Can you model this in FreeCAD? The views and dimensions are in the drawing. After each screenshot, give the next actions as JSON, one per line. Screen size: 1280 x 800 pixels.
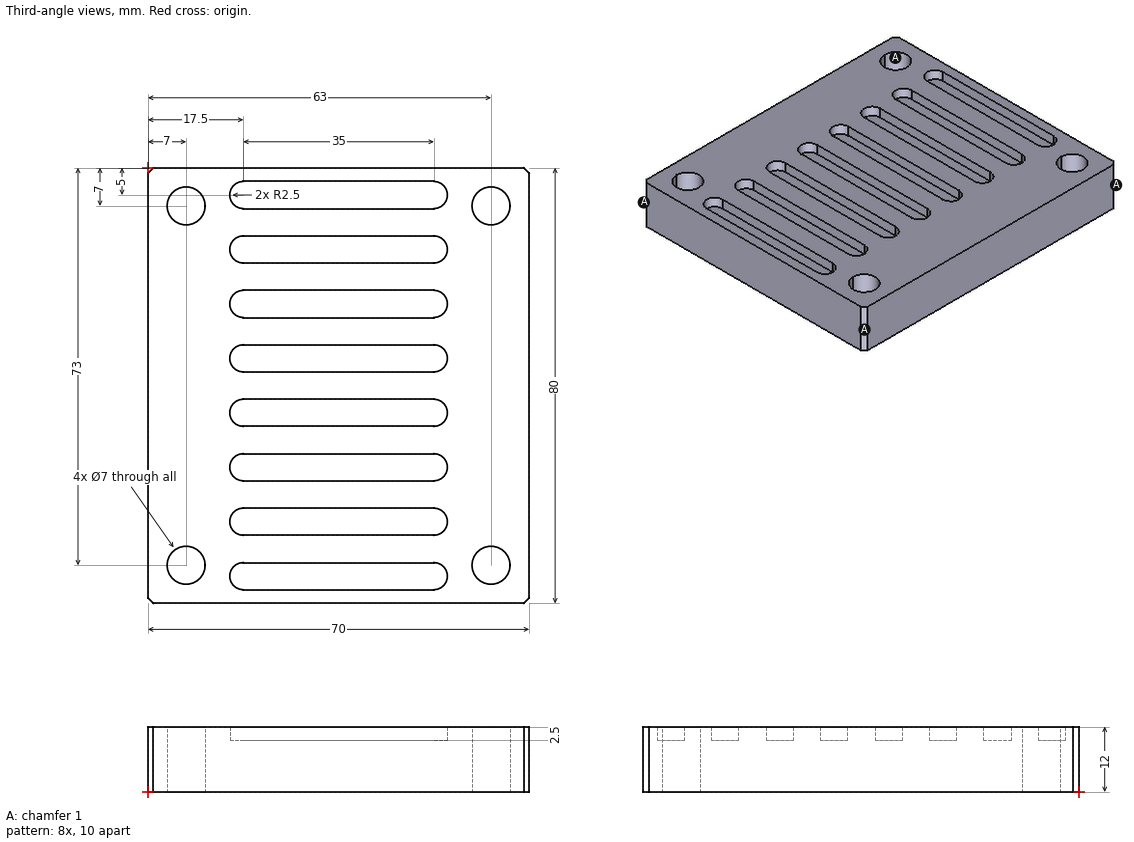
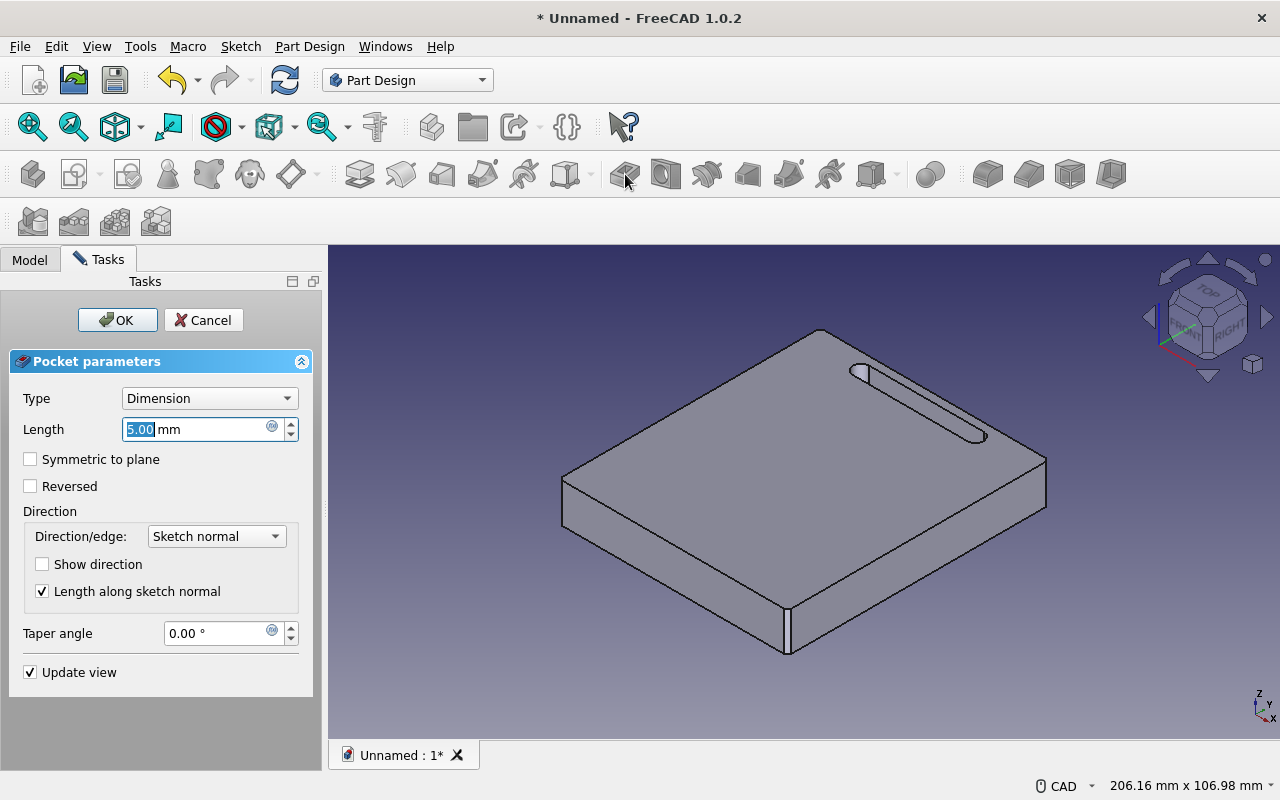
{"action": "type", "text": "2.5"}
{"action": "key", "text": "Tab"}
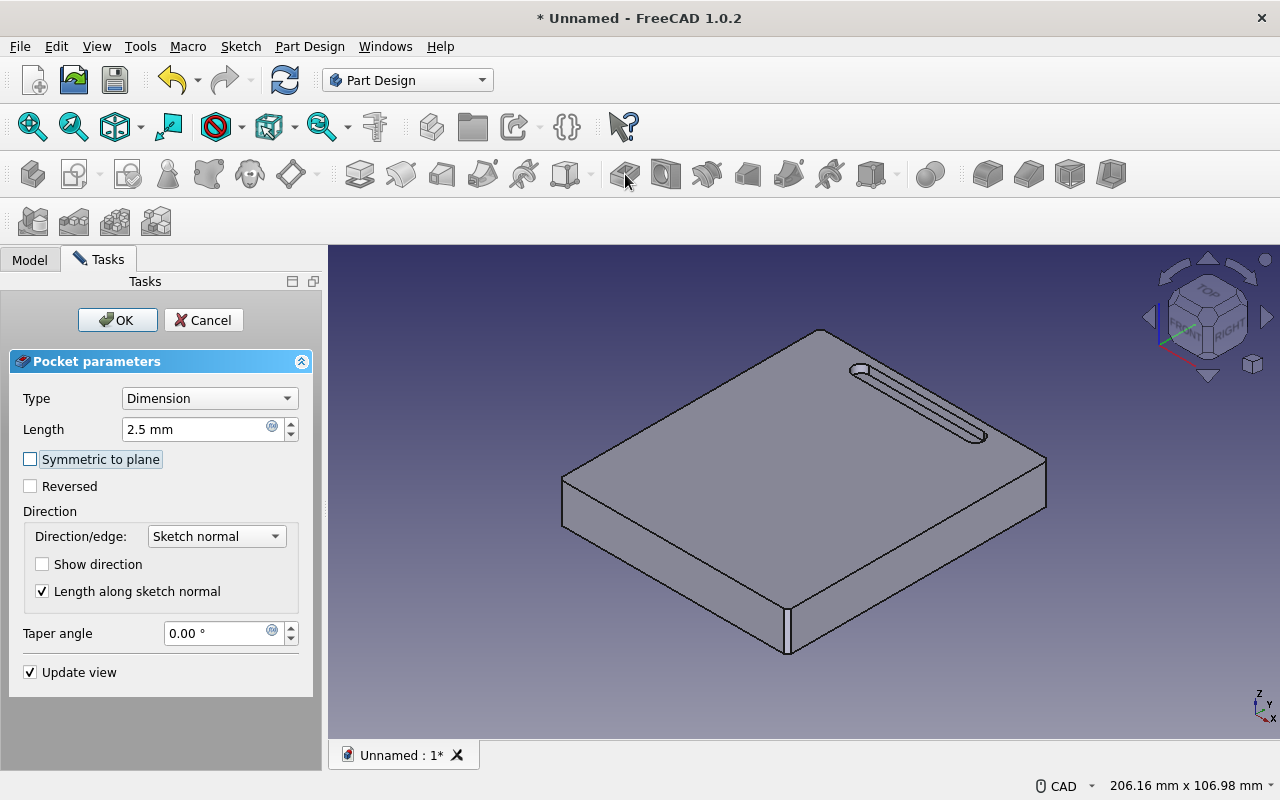
{"action": "left_click", "coordinate": [118, 320]}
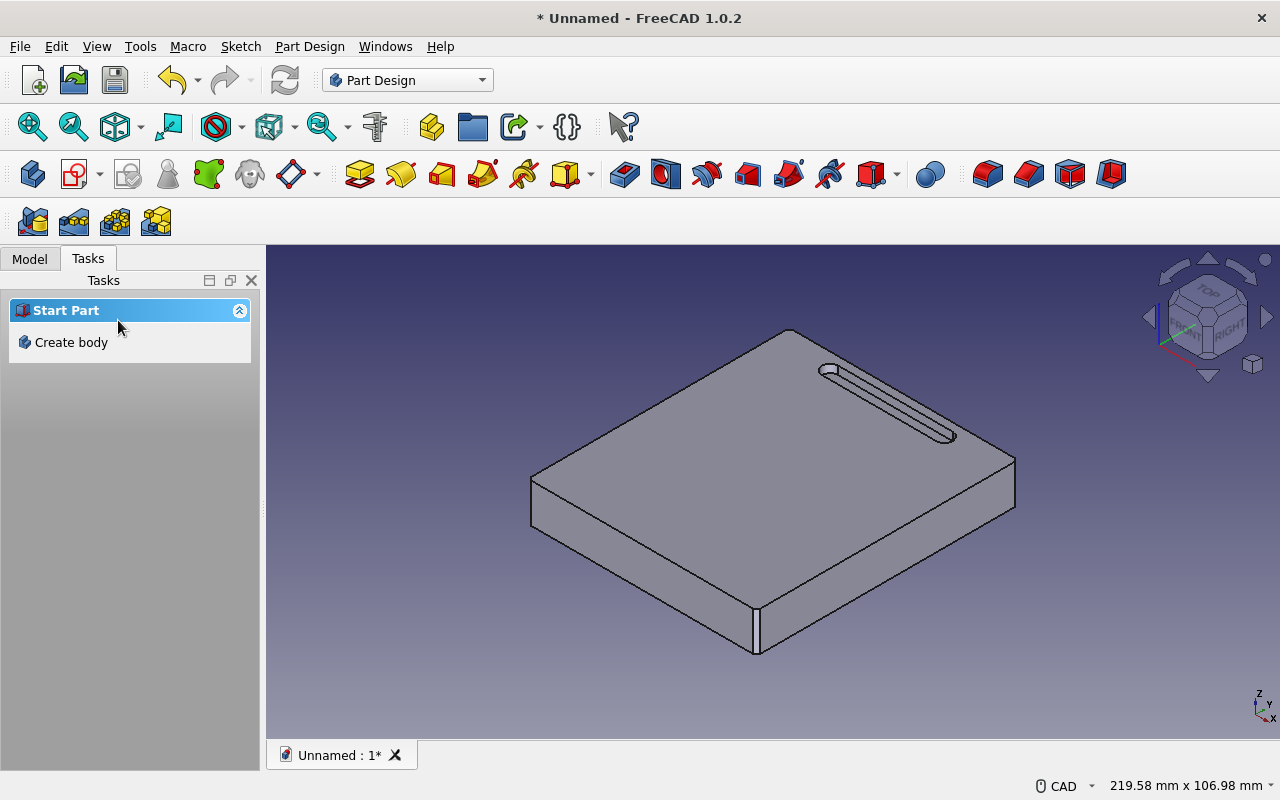
{"action": "left_click", "coordinate": [30, 258]}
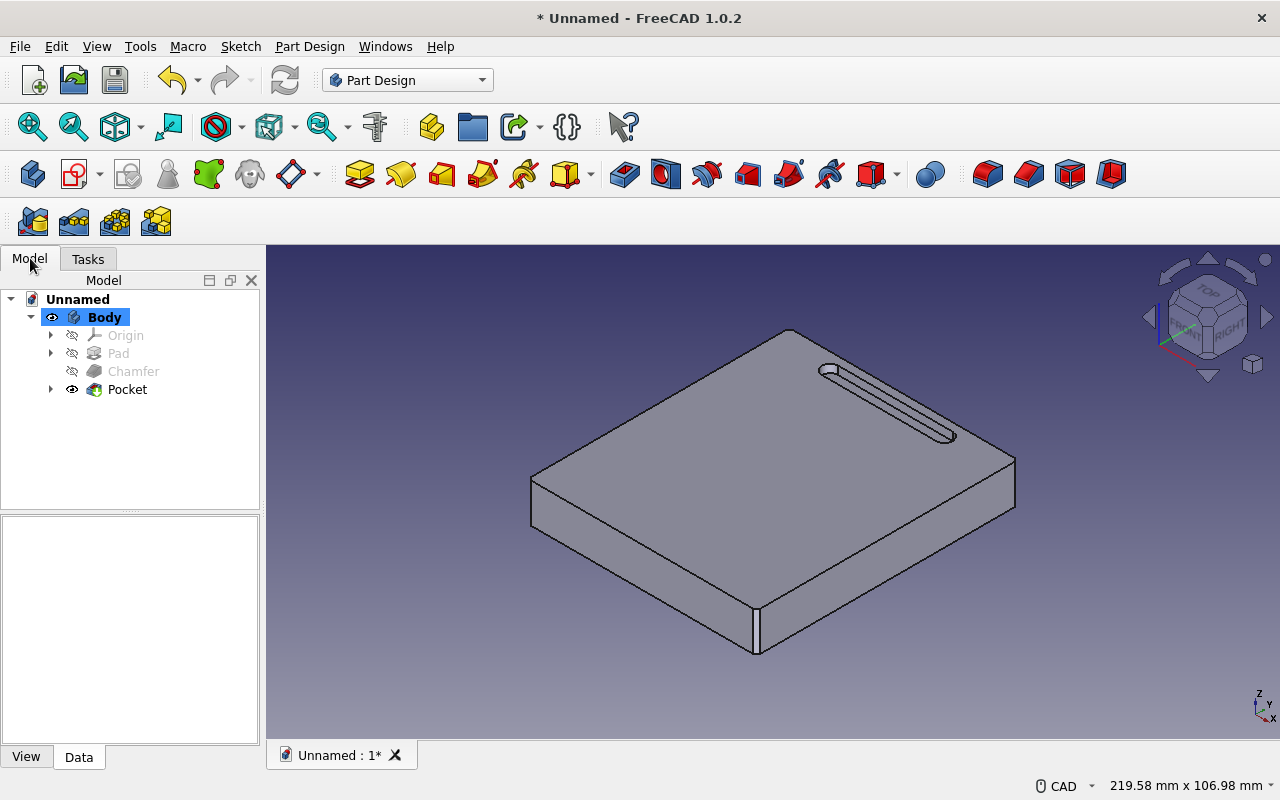
{"action": "left_click", "coordinate": [117, 389]}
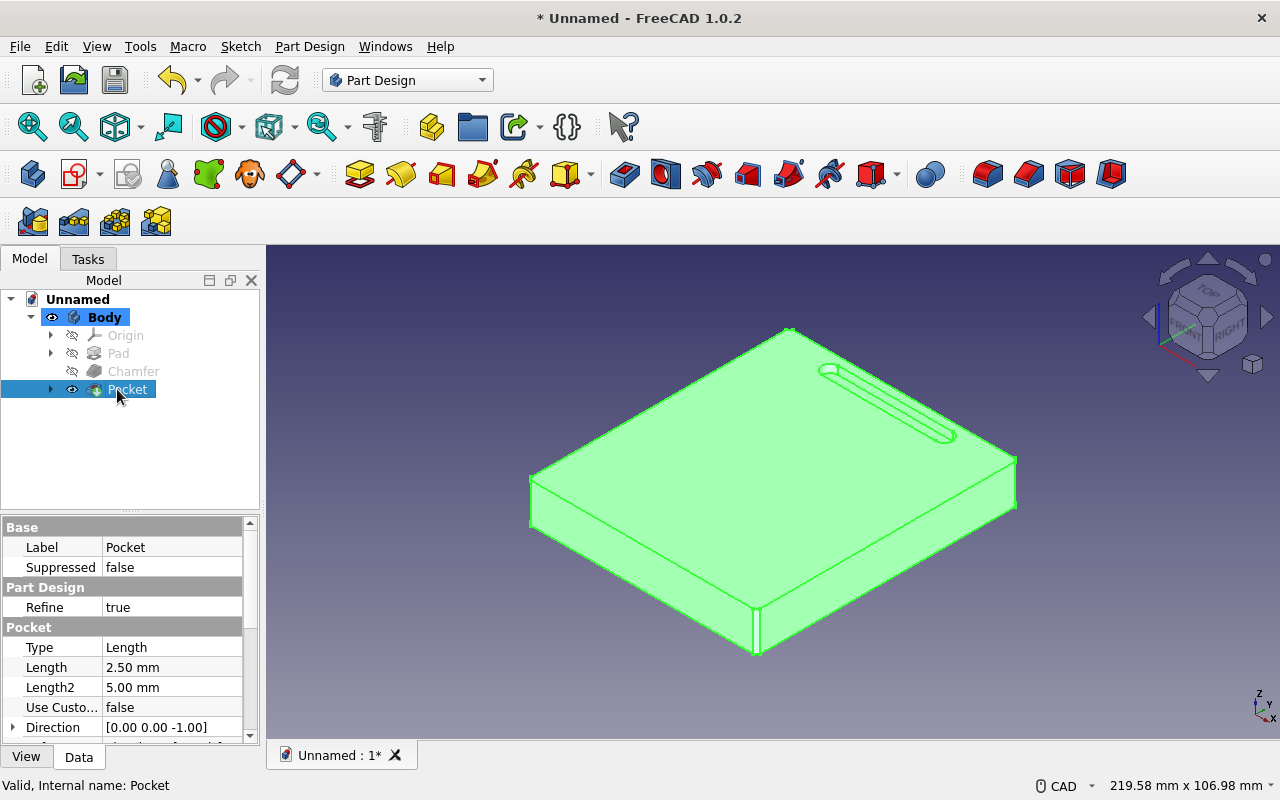
{"action": "left_click", "coordinate": [74, 222]}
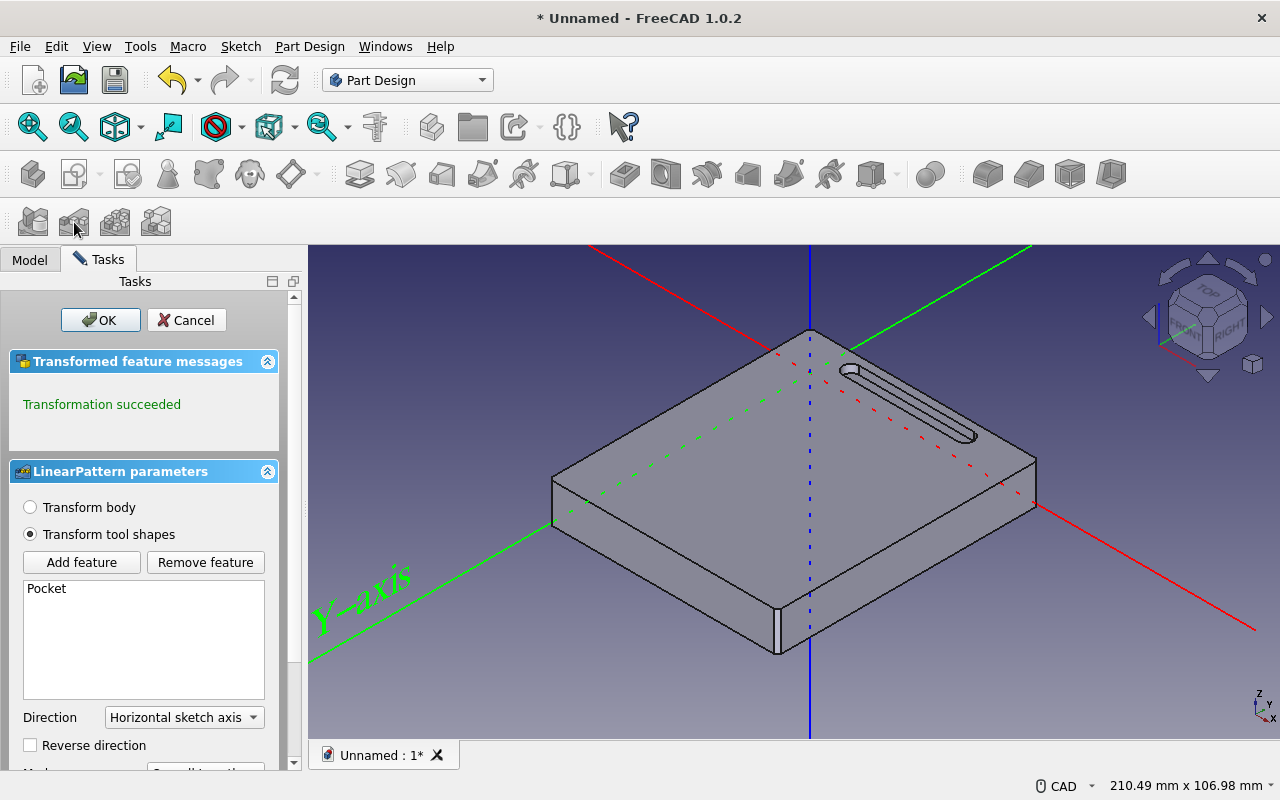
{"action": "left_click", "coordinate": [185, 718]}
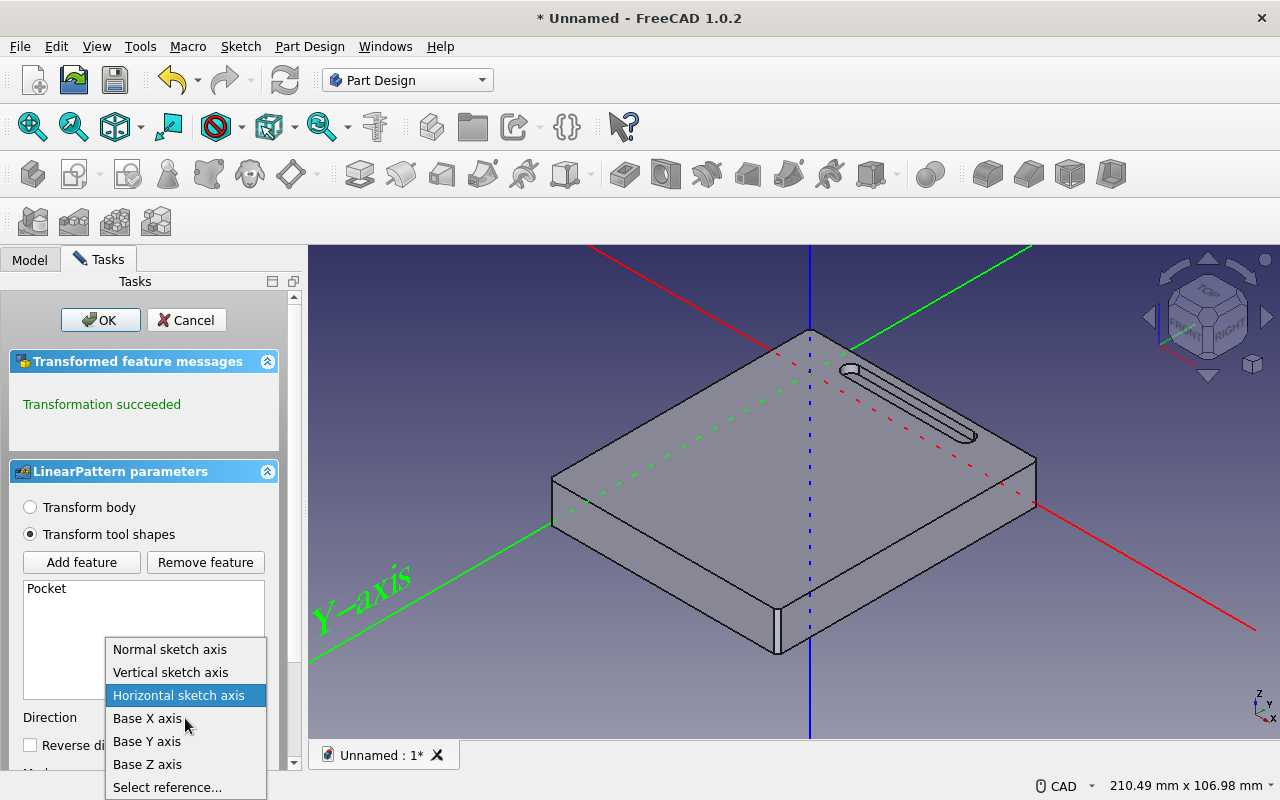
{"action": "left_click", "coordinate": [184, 742]}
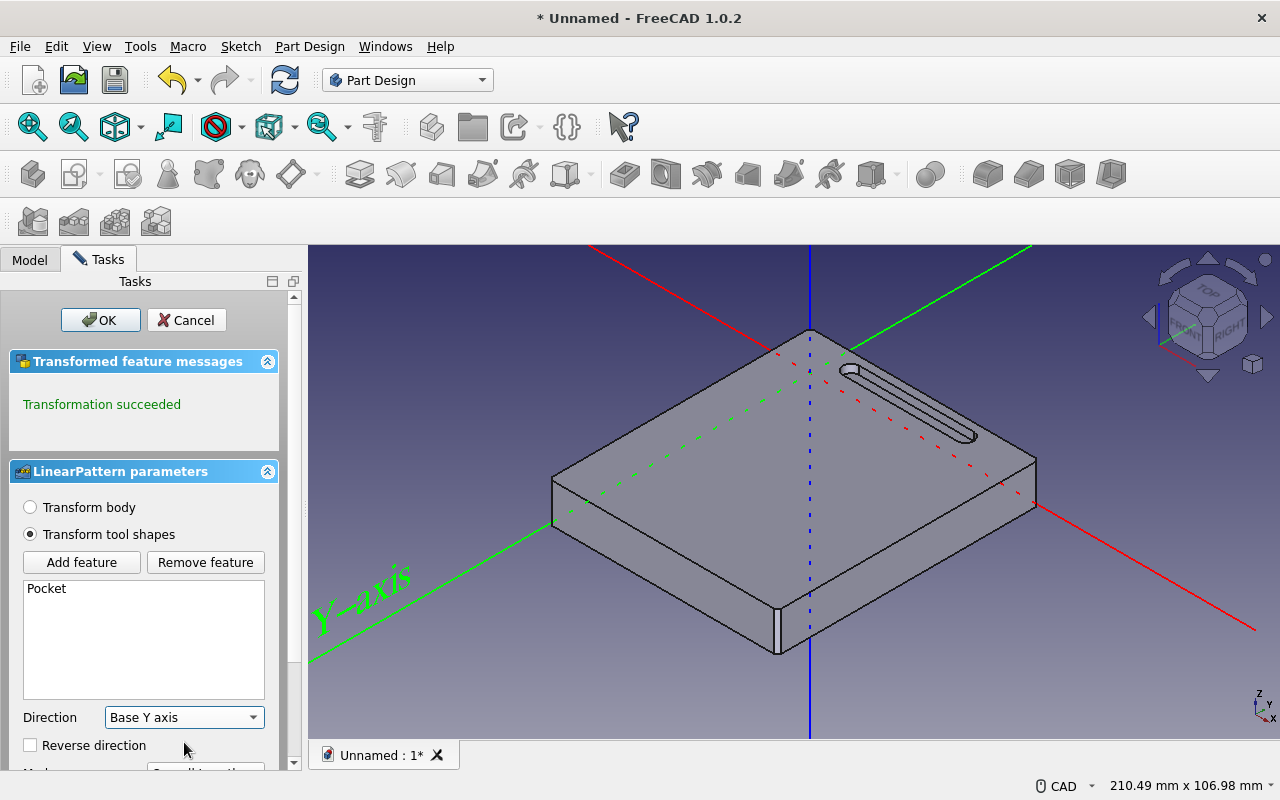
{"action": "scroll", "coordinate": [294, 530], "scroll_direction": "down", "scroll_amount": 2}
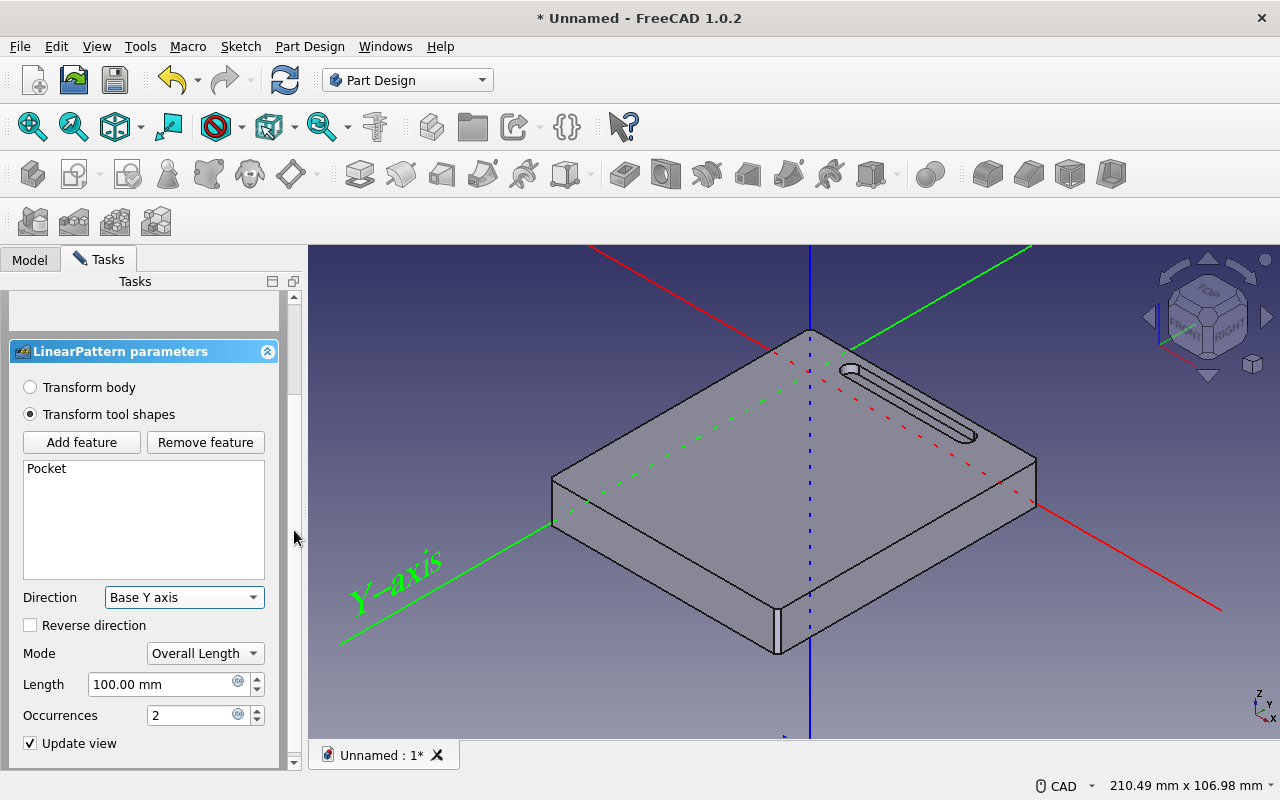
{"action": "left_click", "coordinate": [206, 654]}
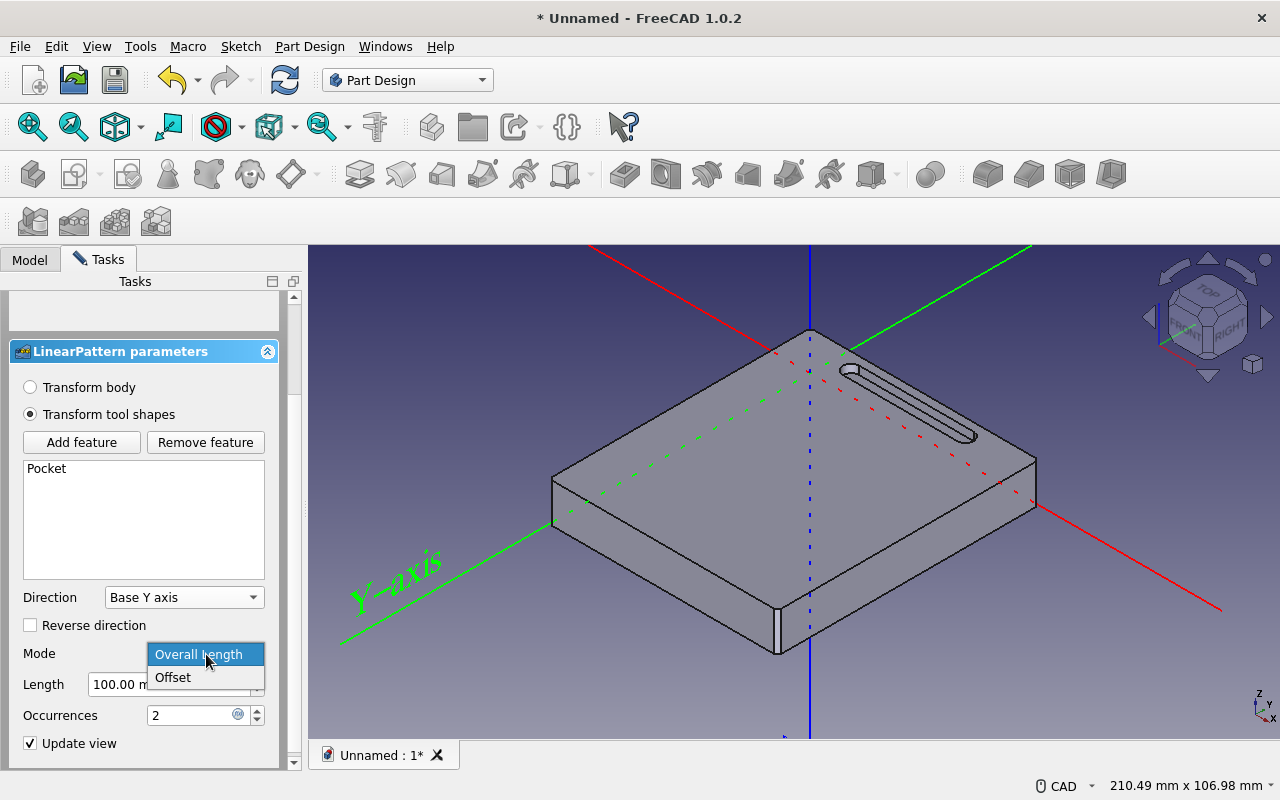
{"action": "left_click", "coordinate": [204, 678]}